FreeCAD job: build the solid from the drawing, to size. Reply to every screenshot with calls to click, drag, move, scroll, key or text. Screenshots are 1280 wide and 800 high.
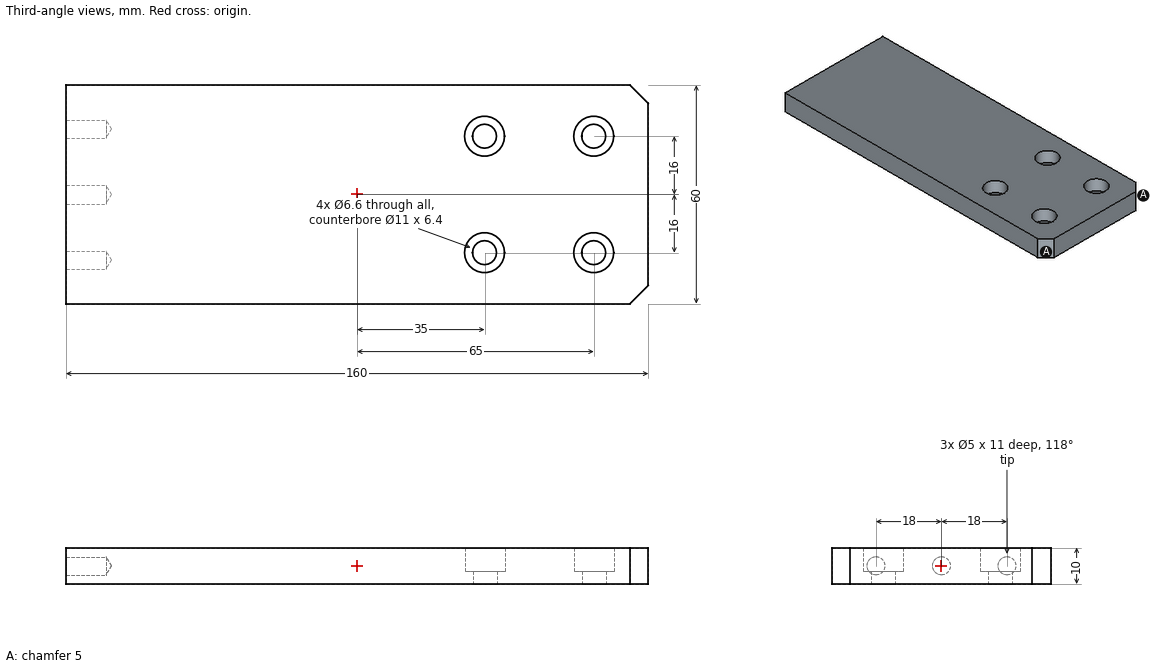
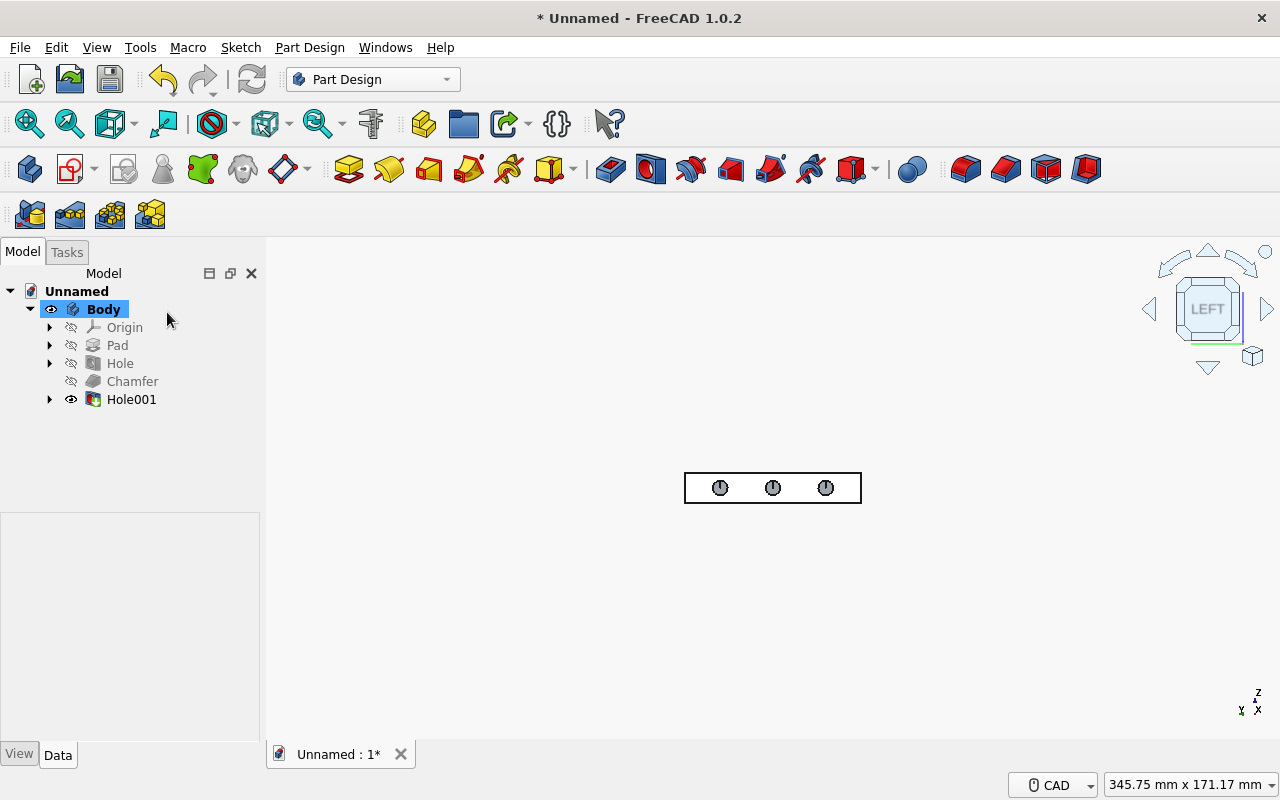
key(0)